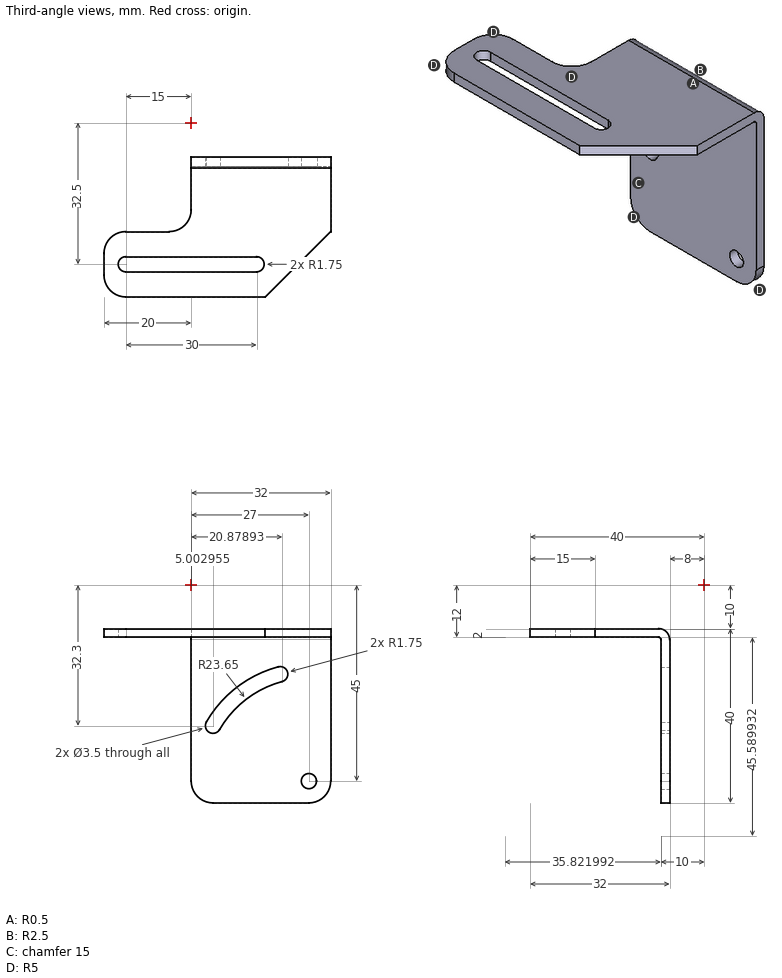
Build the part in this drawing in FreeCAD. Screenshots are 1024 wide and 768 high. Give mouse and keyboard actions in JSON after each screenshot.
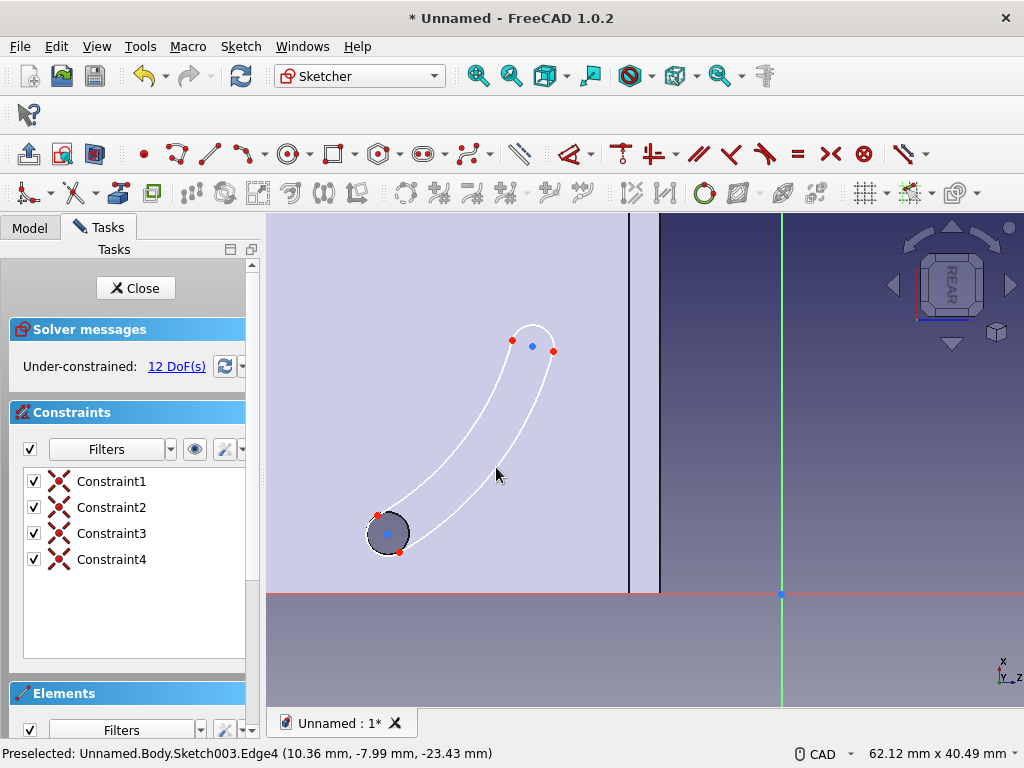
{"action": "left_click", "coordinate": [549, 333]}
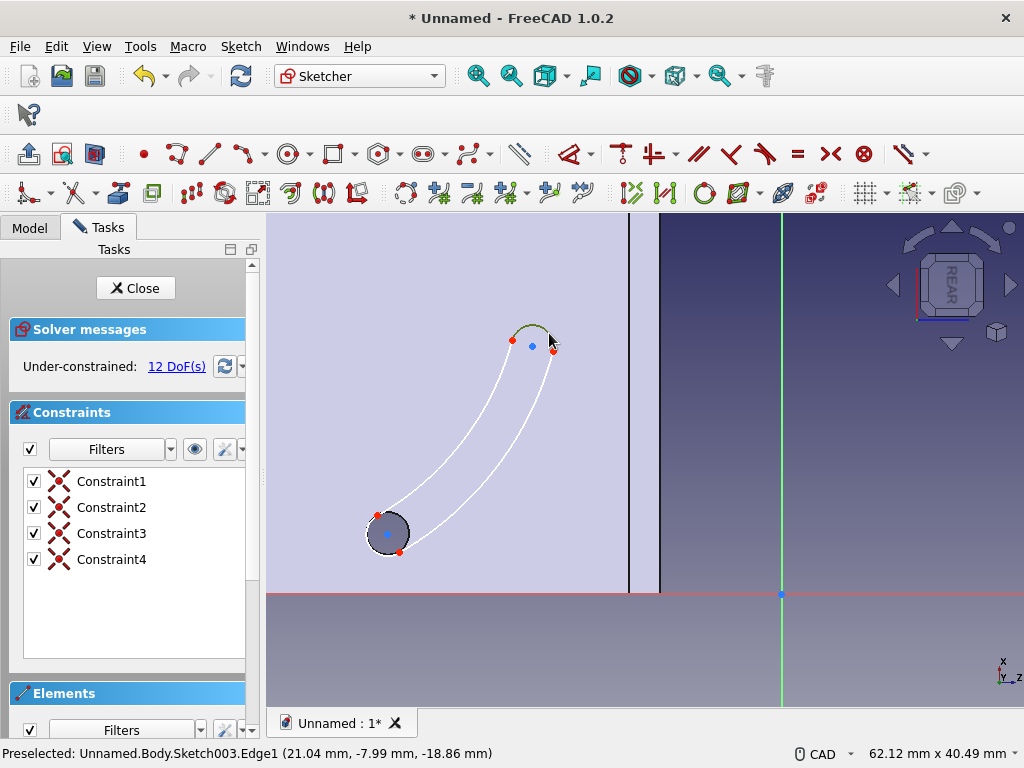
{"action": "left_click", "coordinate": [432, 476]}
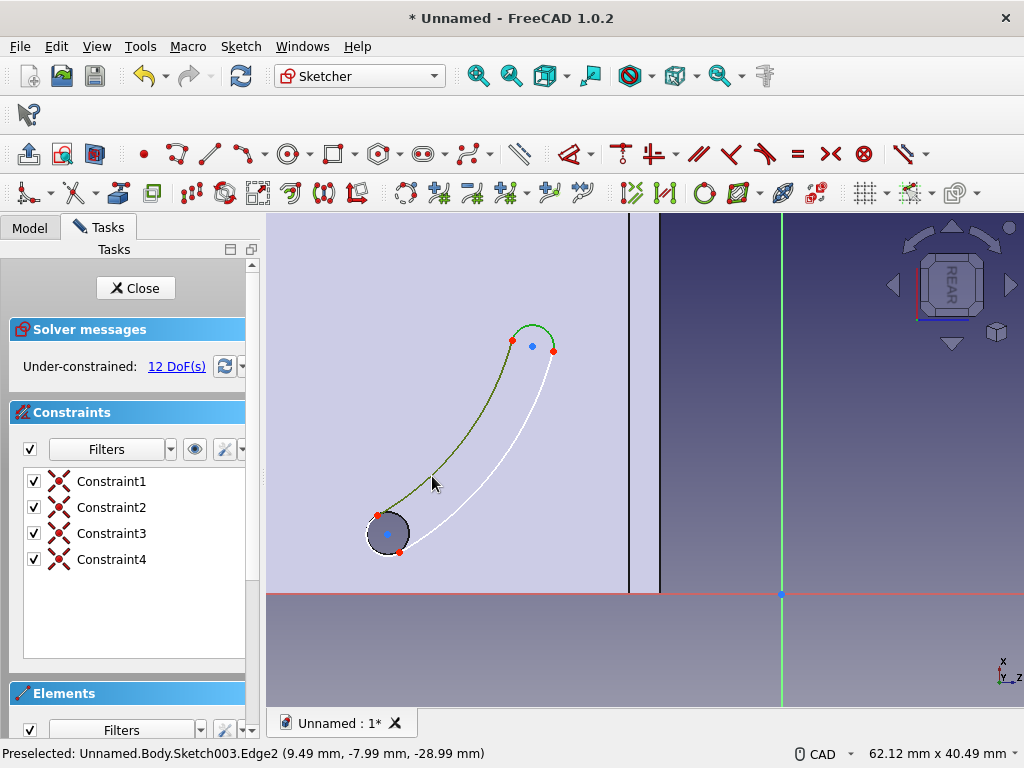
{"action": "key", "text": "t"}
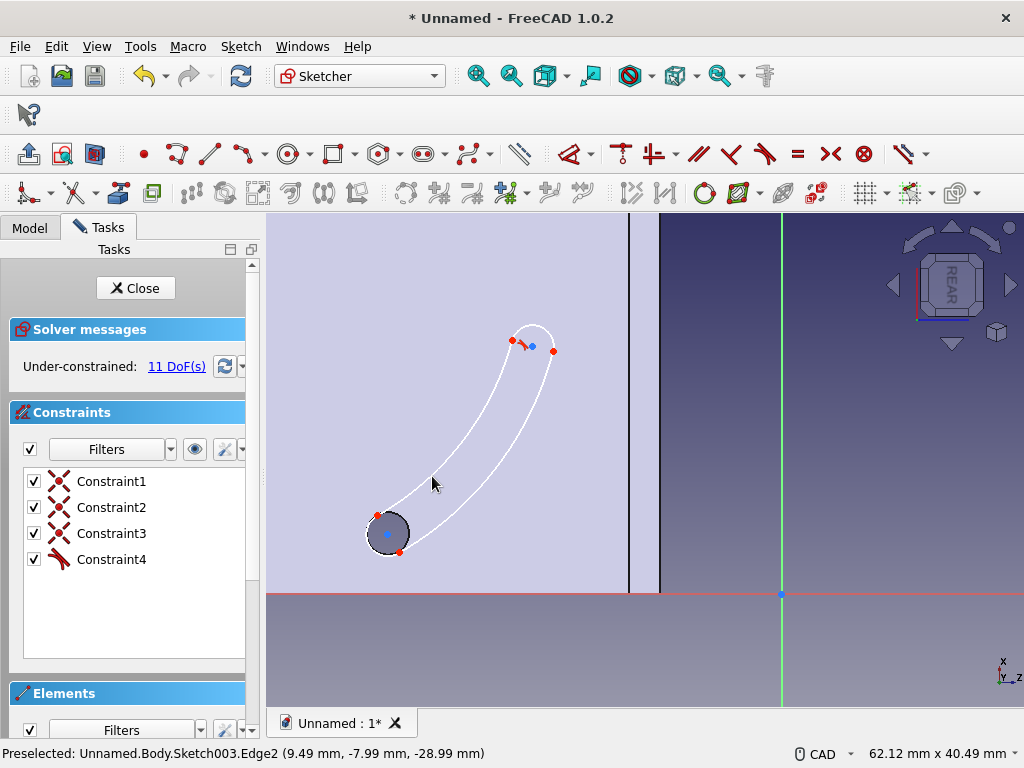
{"action": "left_click", "coordinate": [549, 333]}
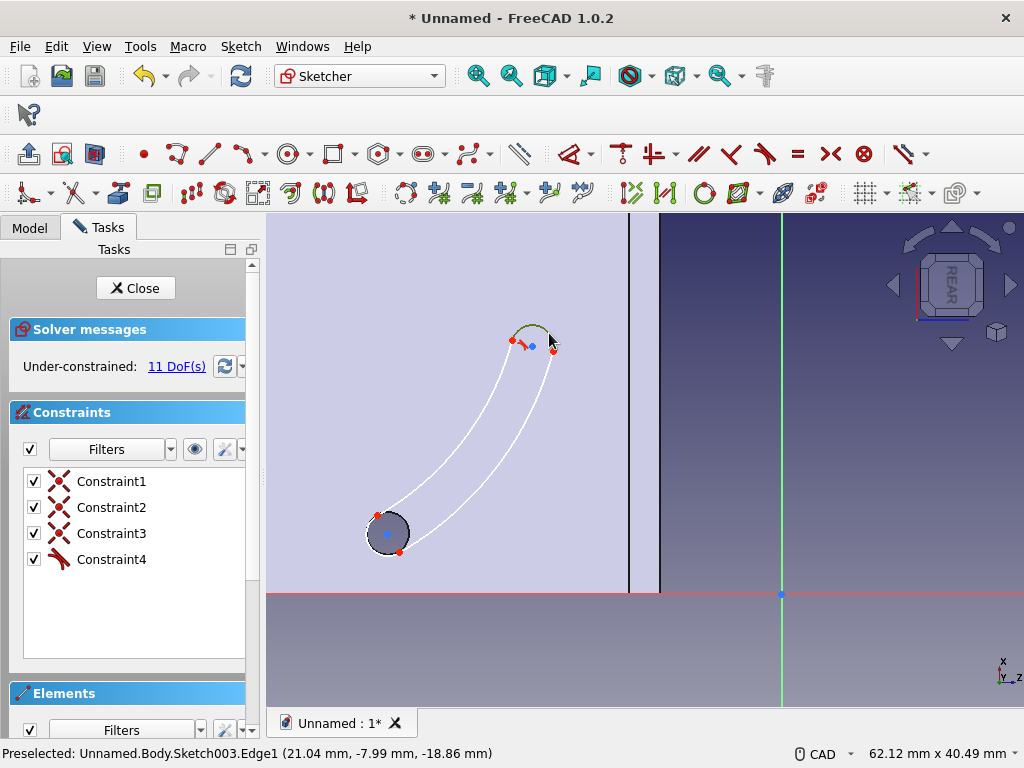
{"action": "left_click", "coordinate": [461, 506]}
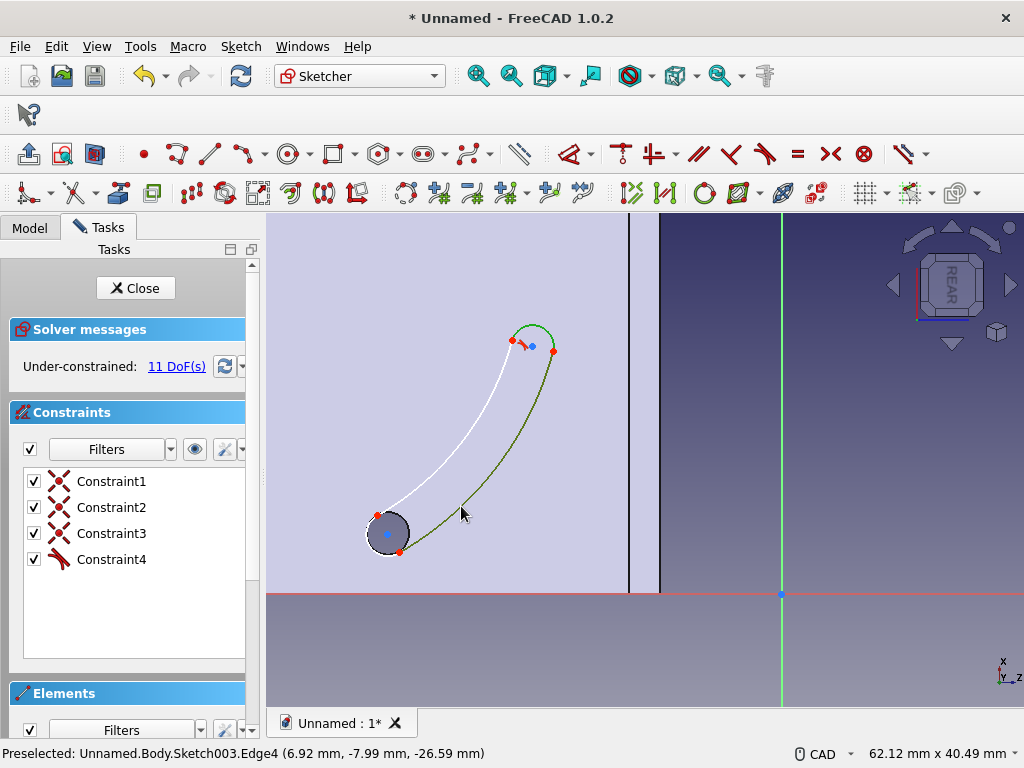
{"action": "key", "text": "t"}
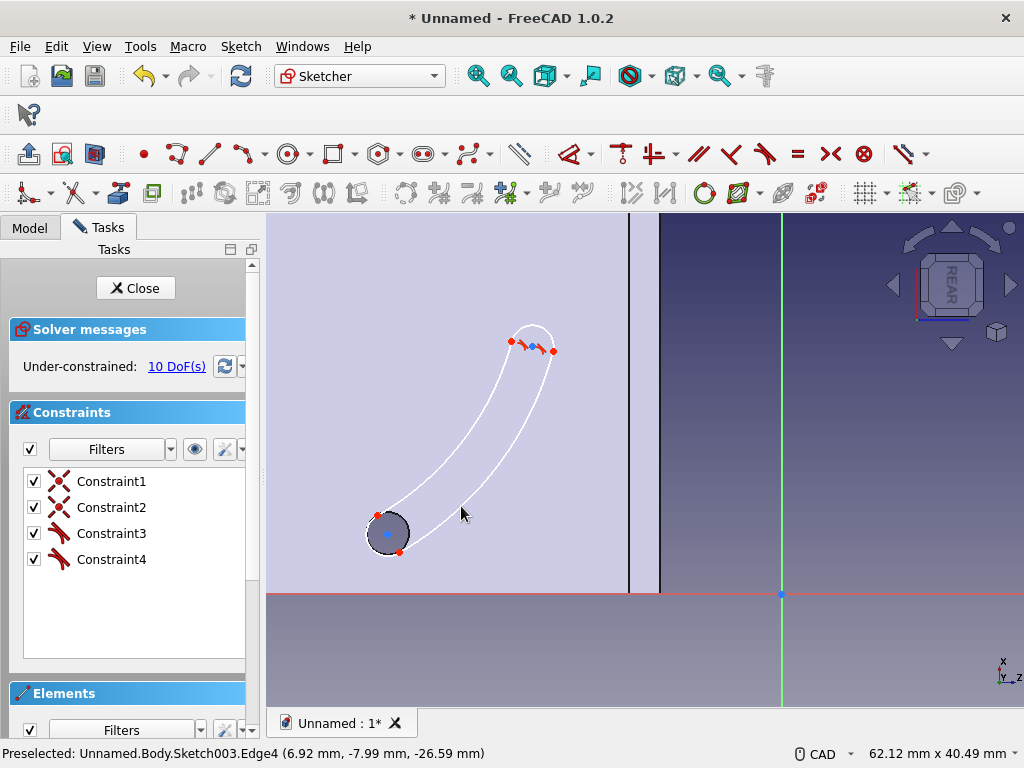
{"action": "left_click", "coordinate": [432, 476]}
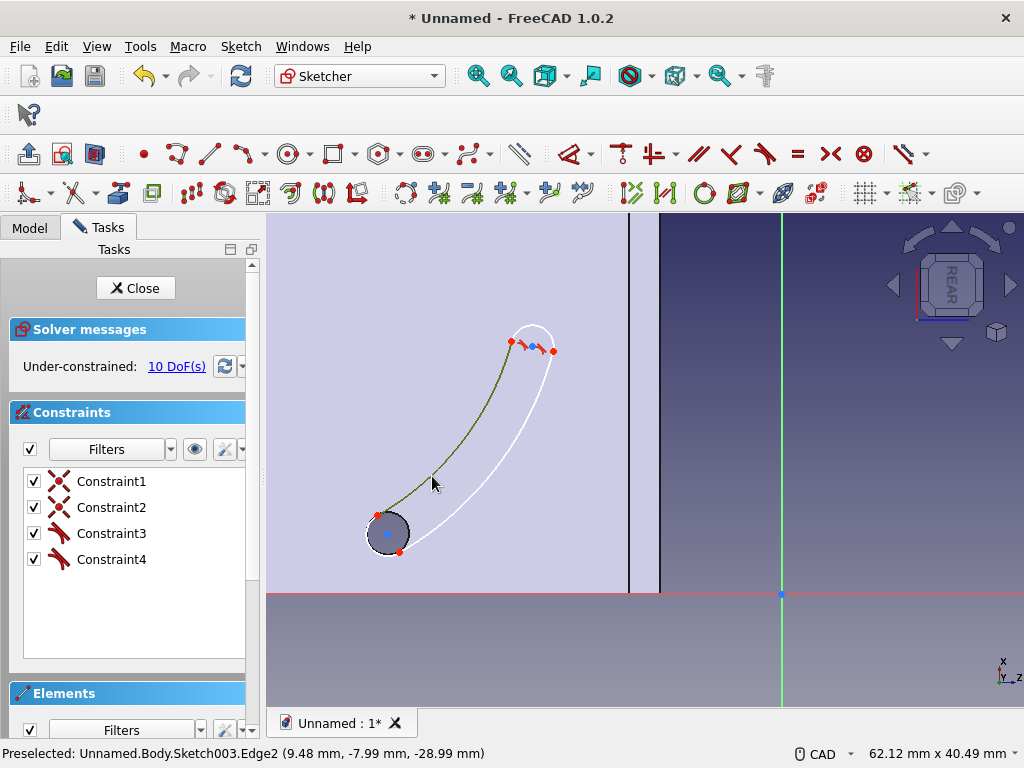
{"action": "left_click", "coordinate": [366, 533]}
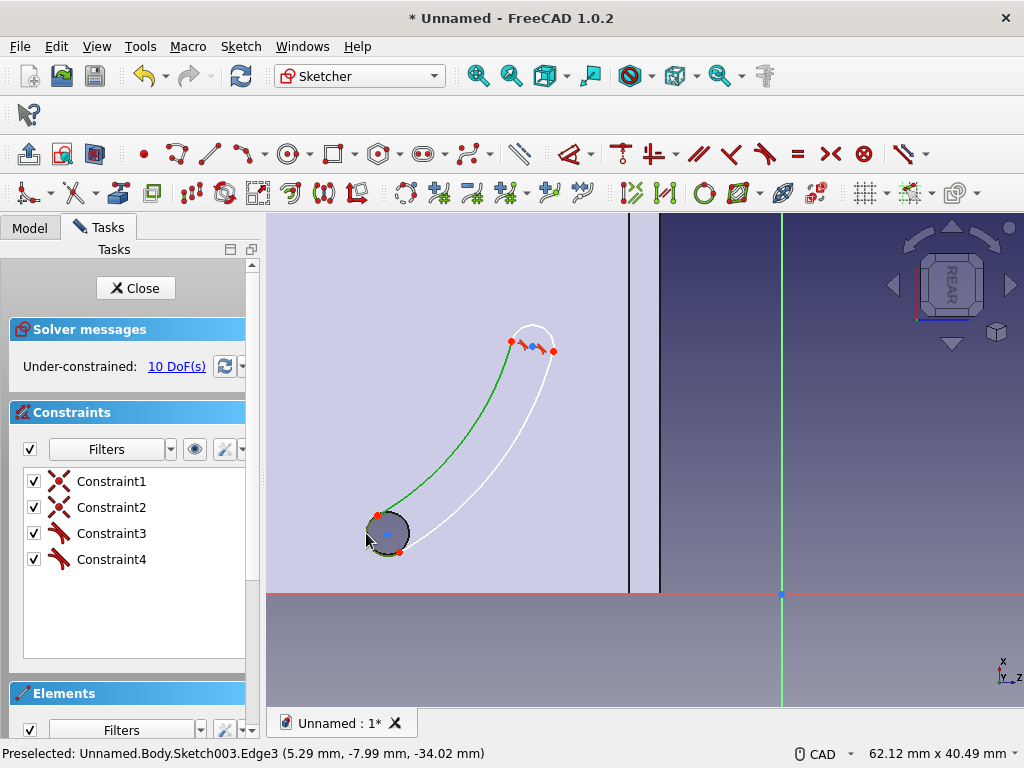
{"action": "key", "text": "t"}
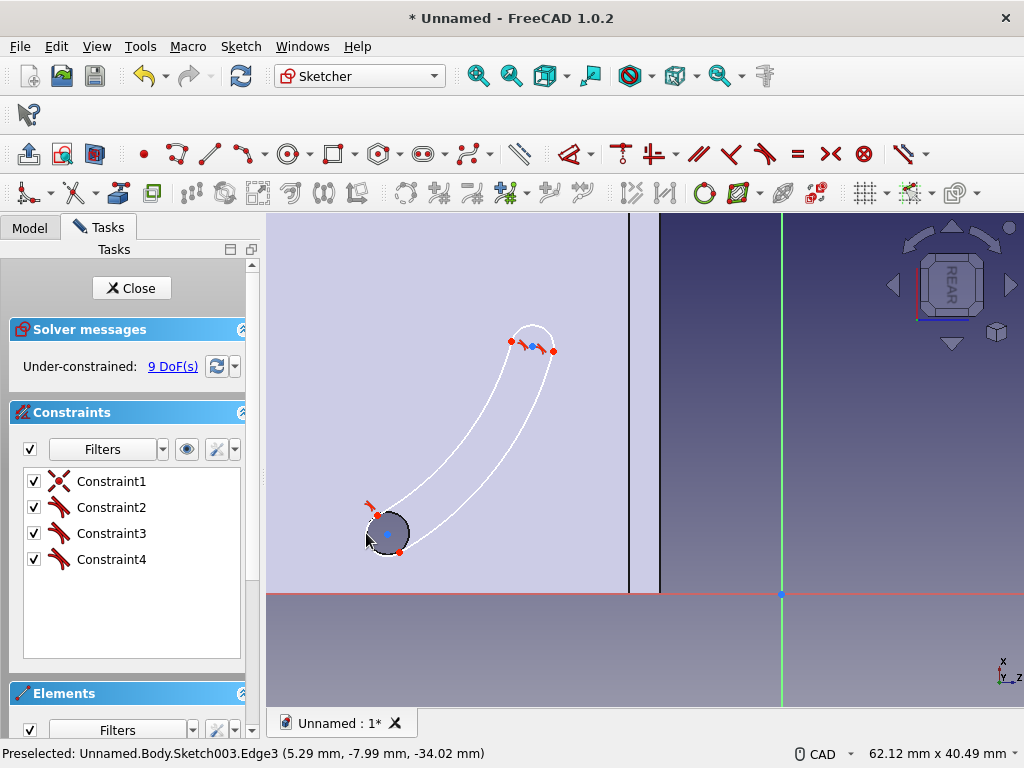
{"action": "left_click", "coordinate": [366, 533]}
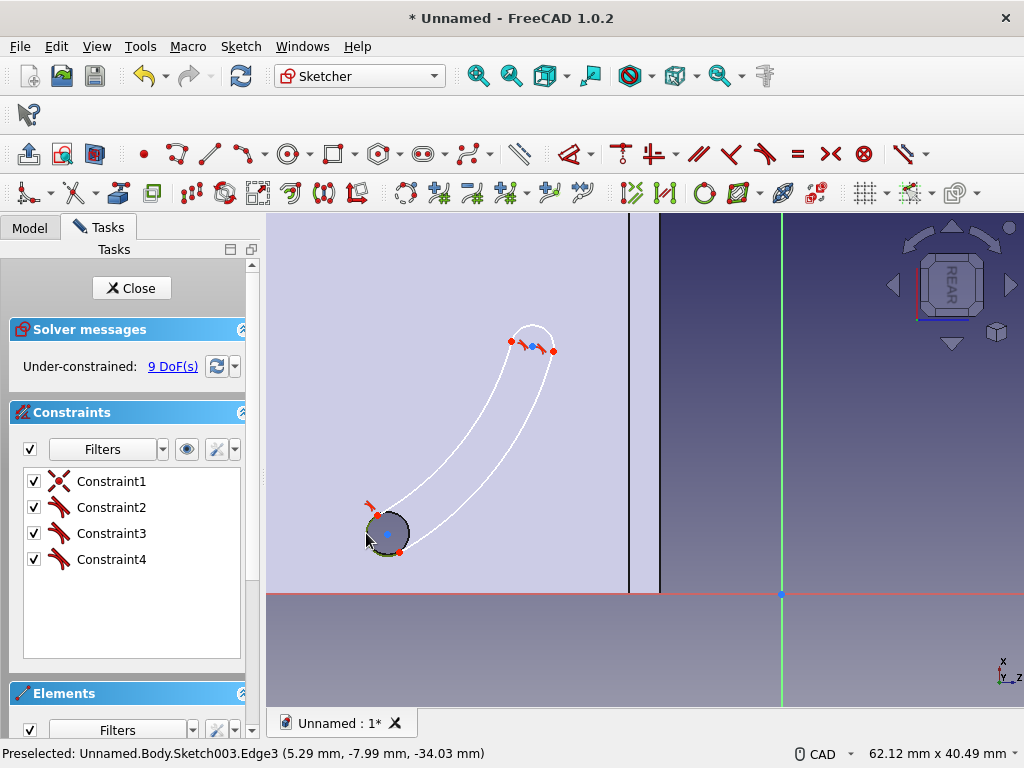
{"action": "left_click", "coordinate": [461, 506]}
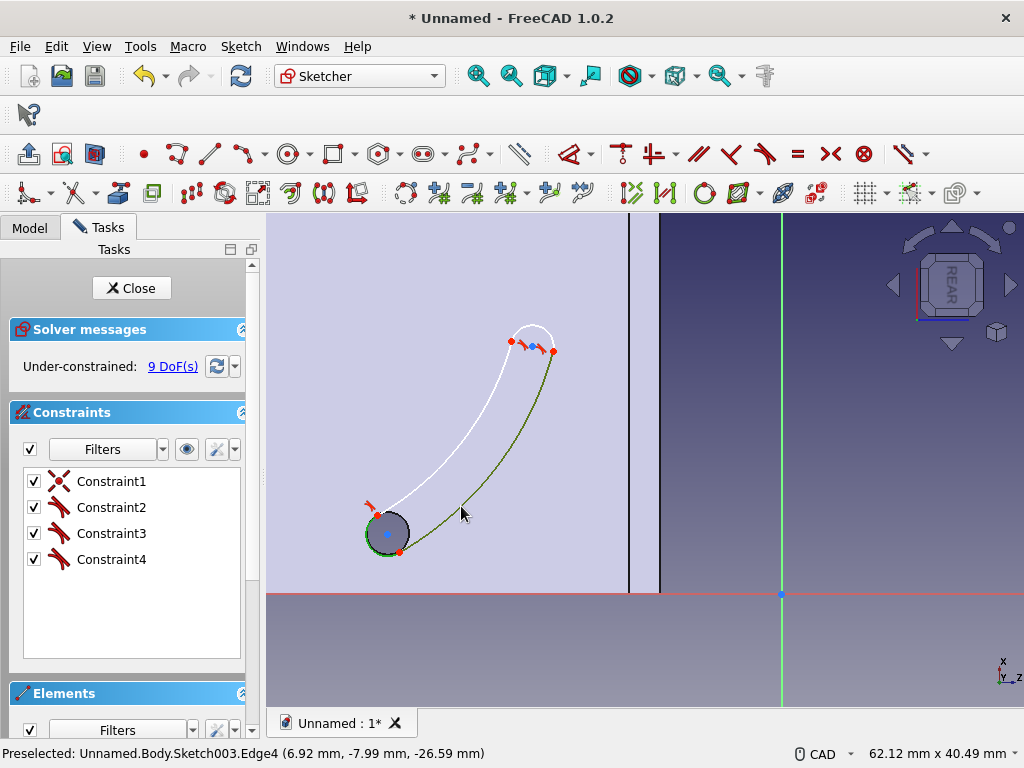
{"action": "left_click", "coordinate": [765, 154]}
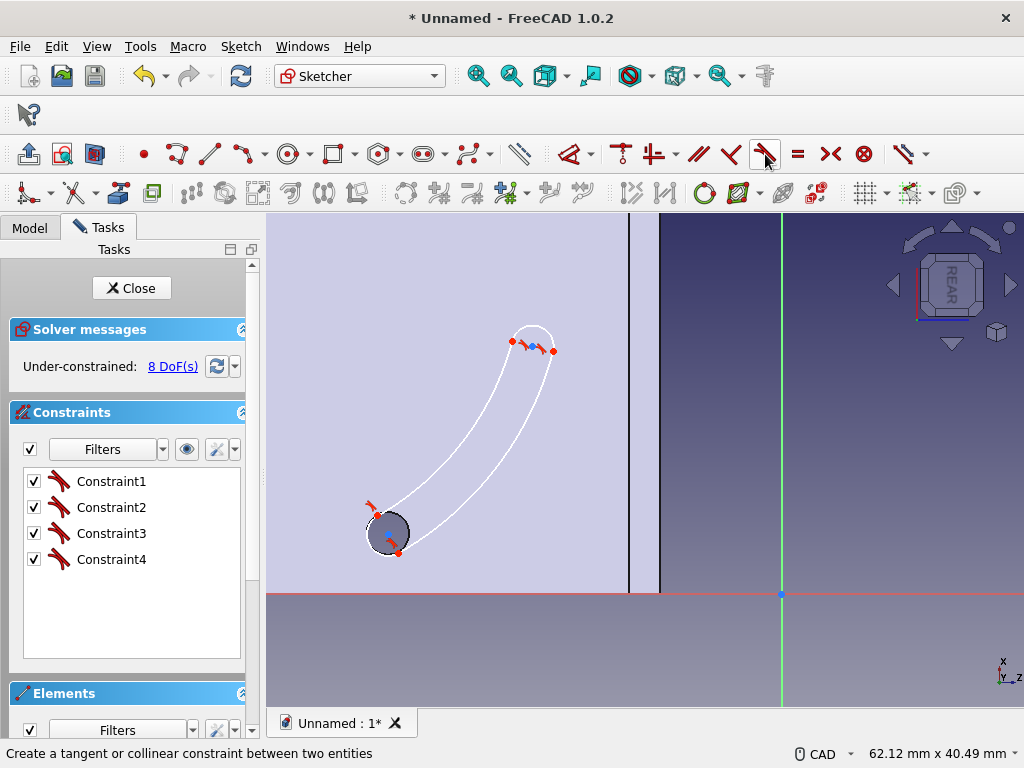
{"action": "left_click", "coordinate": [432, 476]}